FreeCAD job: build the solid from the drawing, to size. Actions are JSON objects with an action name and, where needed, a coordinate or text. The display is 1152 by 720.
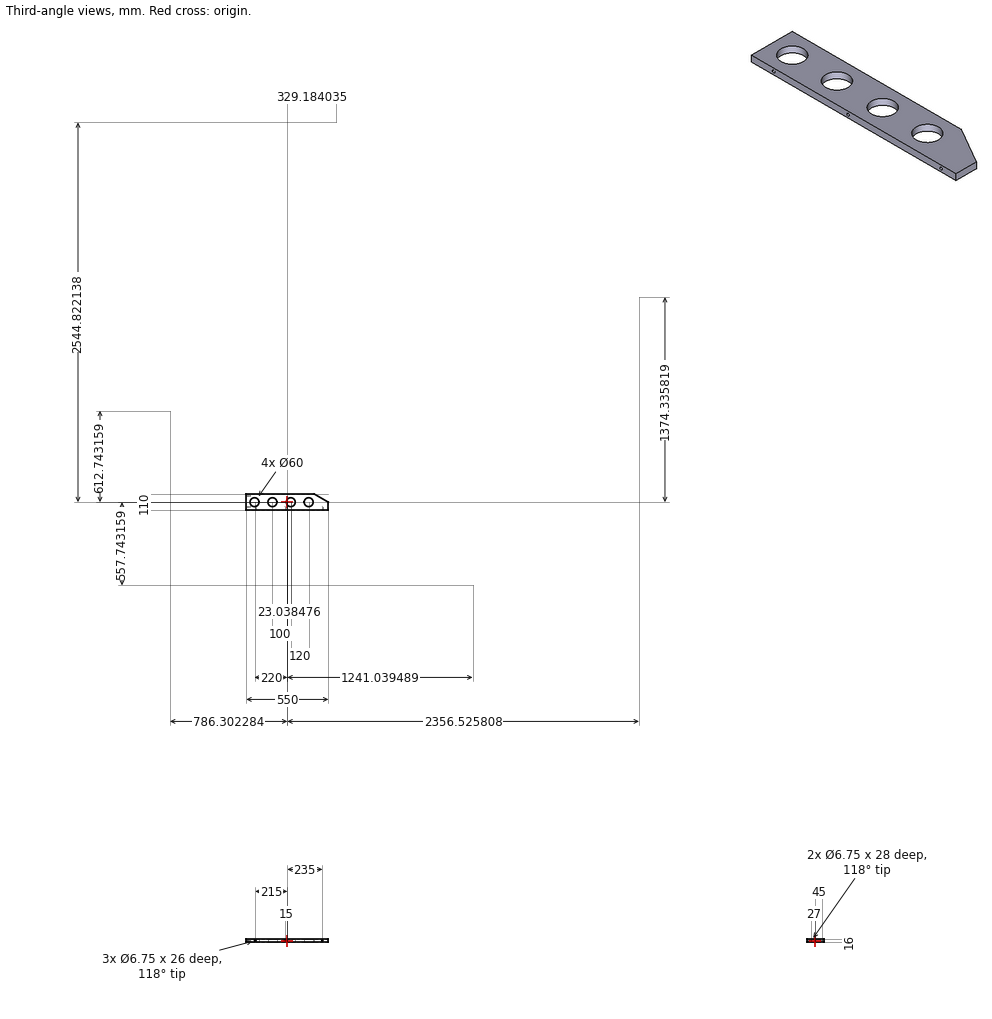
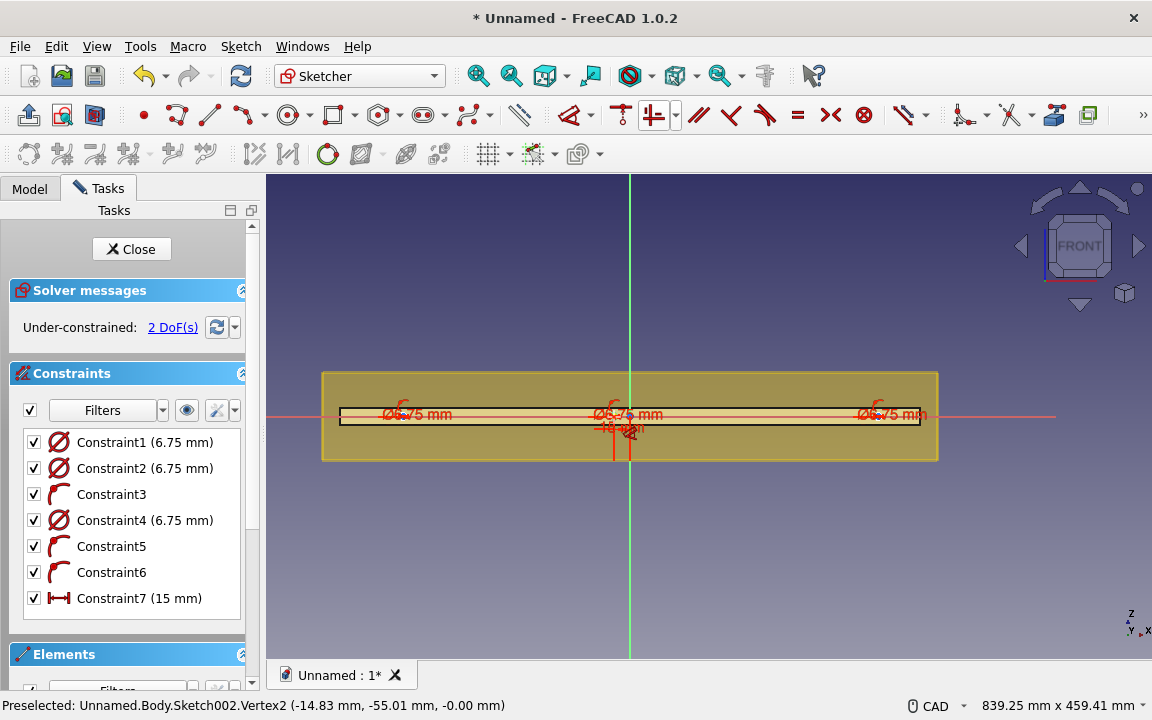
{"action": "left_click", "coordinate": [403, 417]}
{"action": "left_click", "coordinate": [517, 451]}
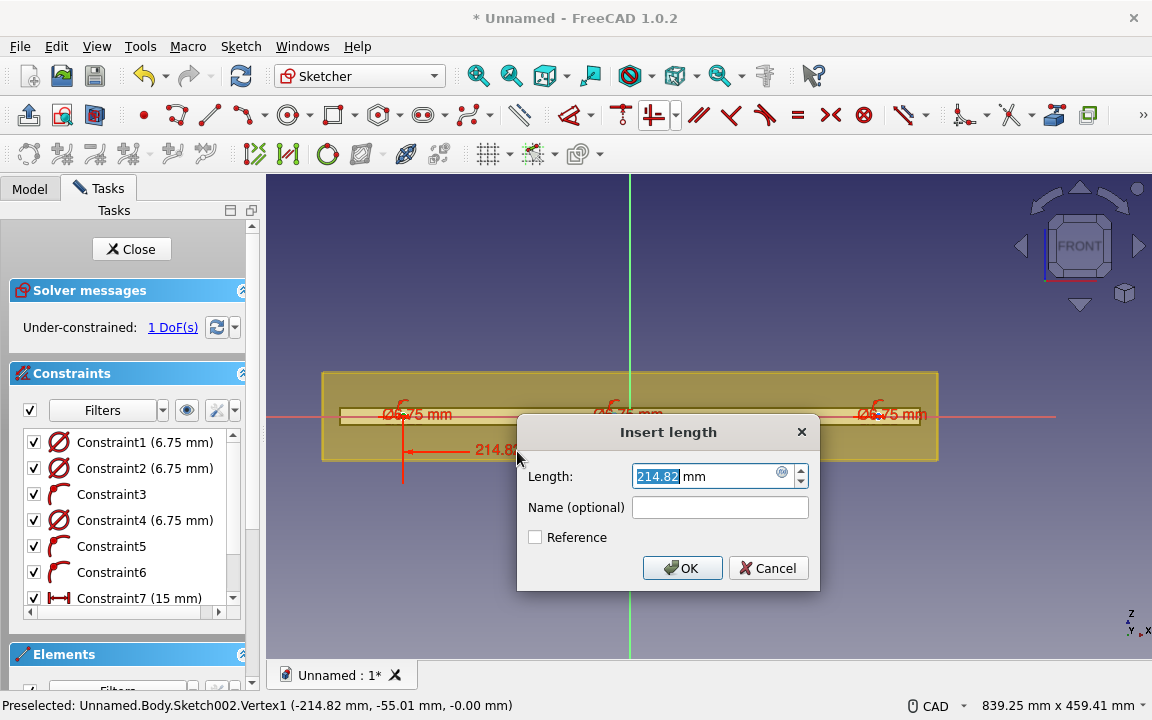
{"action": "type", "text": "215"}
{"action": "key", "text": "Return"}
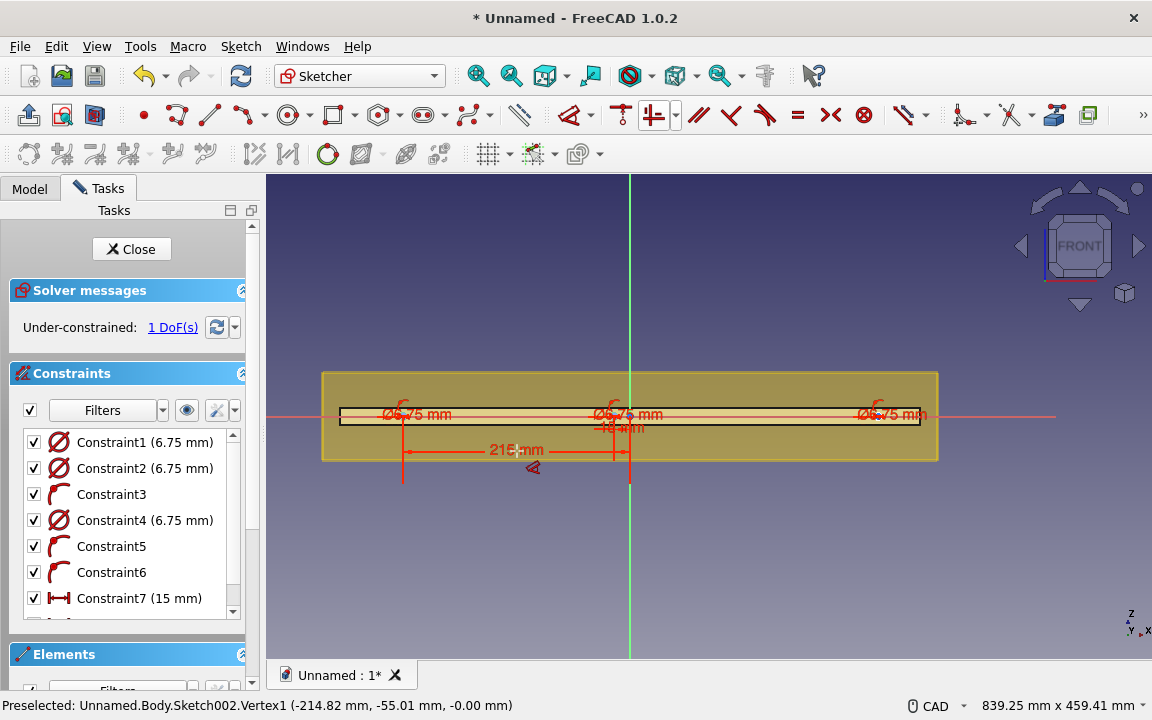
{"action": "left_click", "coordinate": [878, 417]}
{"action": "left_click", "coordinate": [754, 451]}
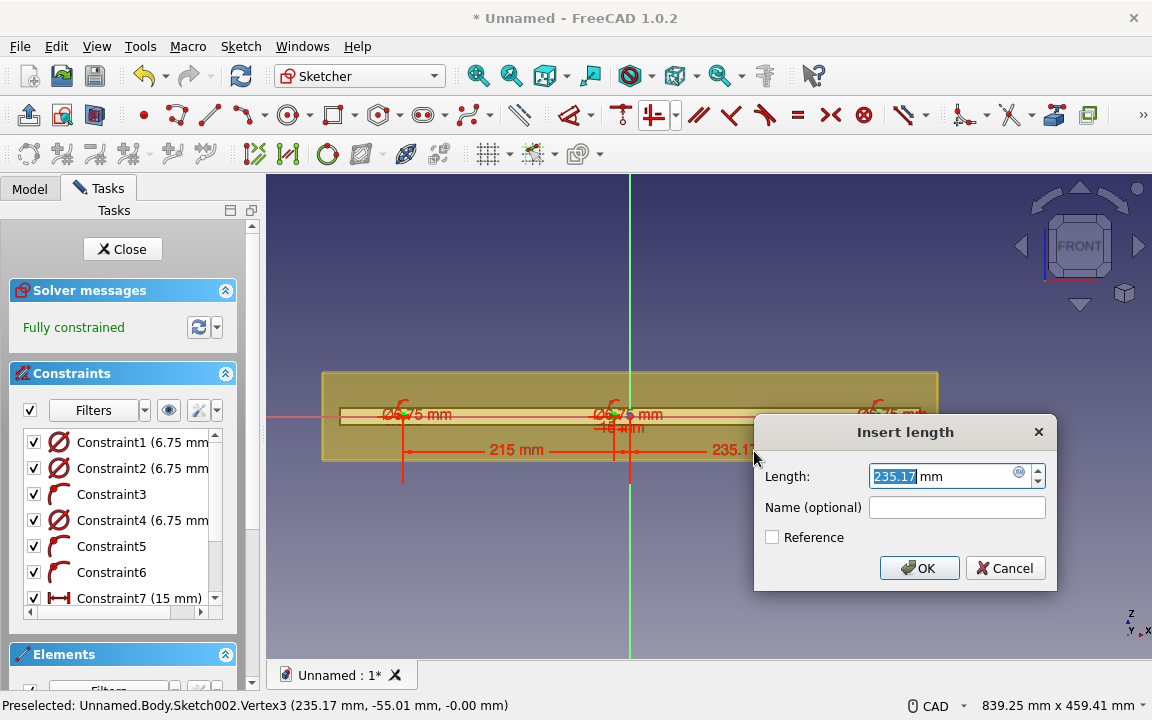
{"action": "type", "text": "235"}
{"action": "key", "text": "Return"}
{"action": "key", "text": "Escape"}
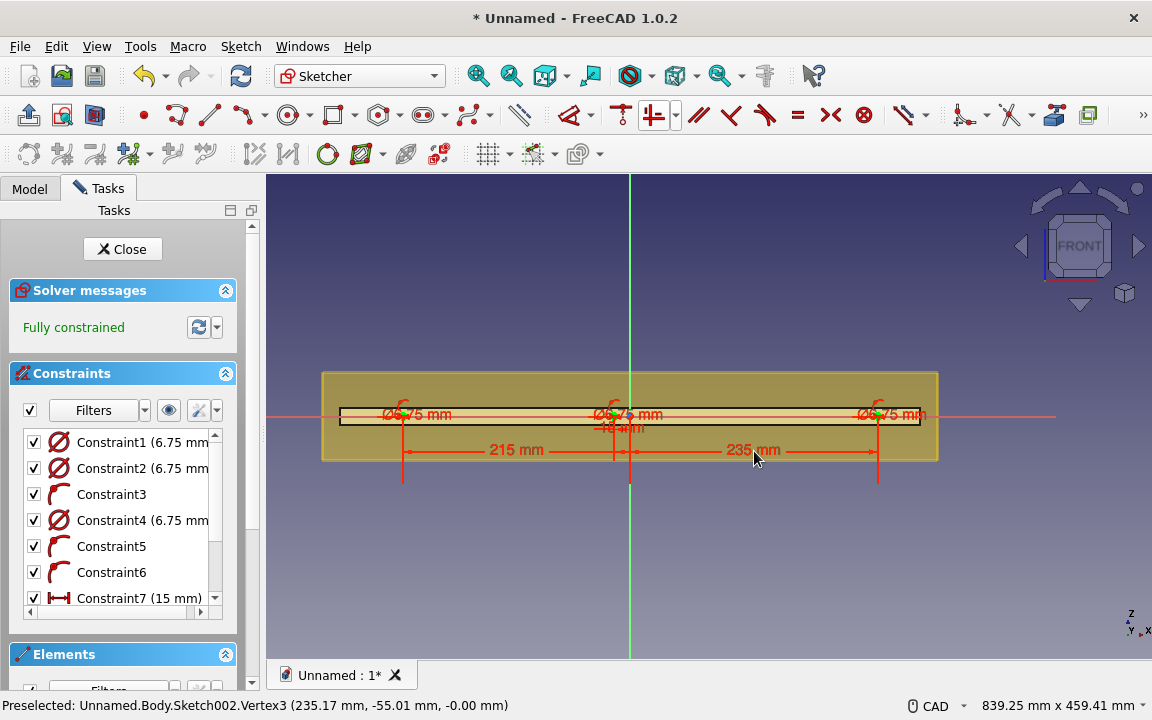
{"action": "left_click", "coordinate": [123, 249]}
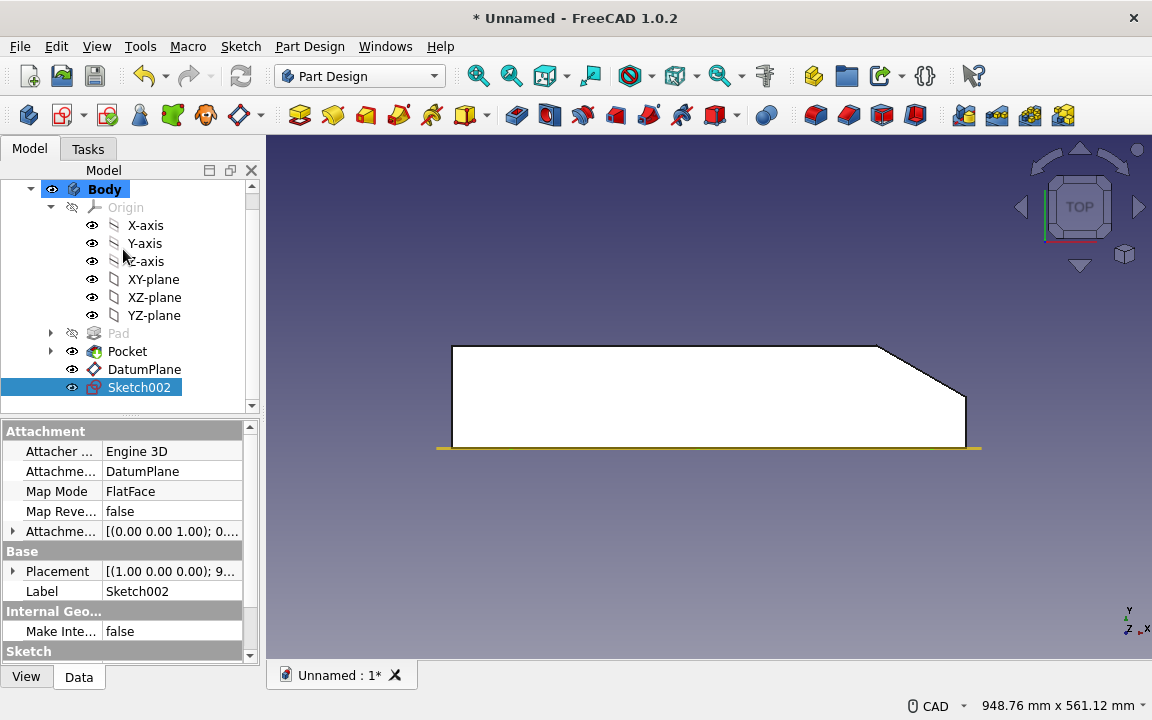
{"action": "left_click", "coordinate": [550, 116]}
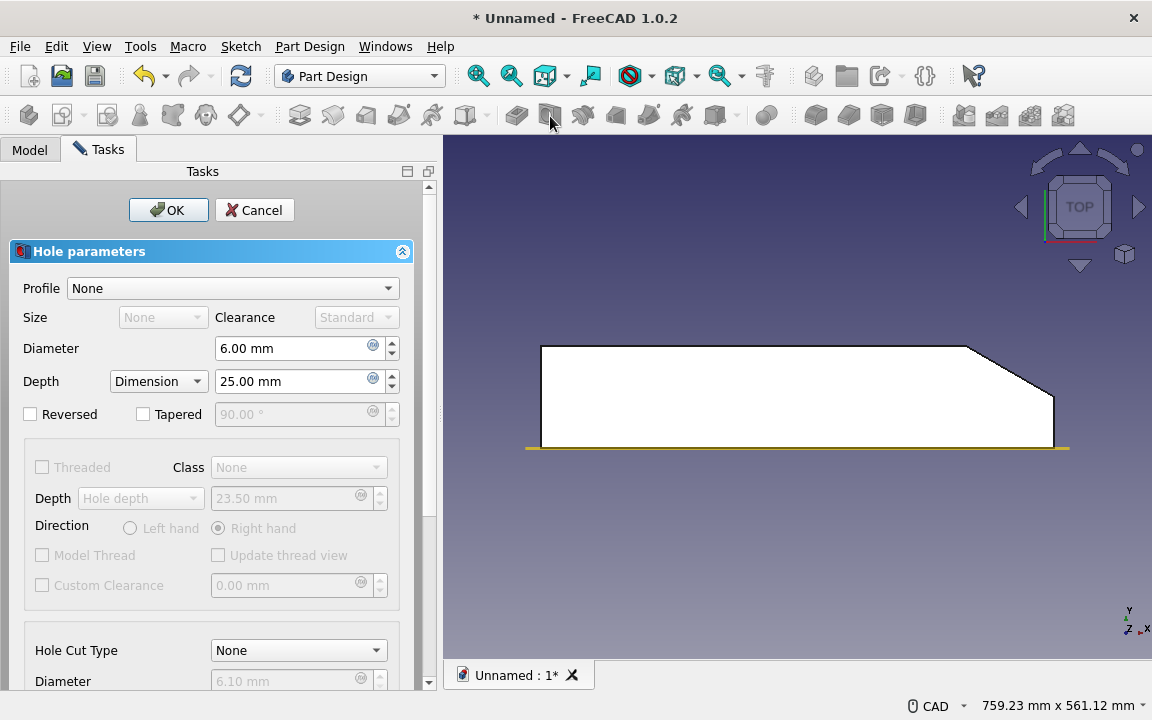
{"action": "triple_click", "coordinate": [300, 348]}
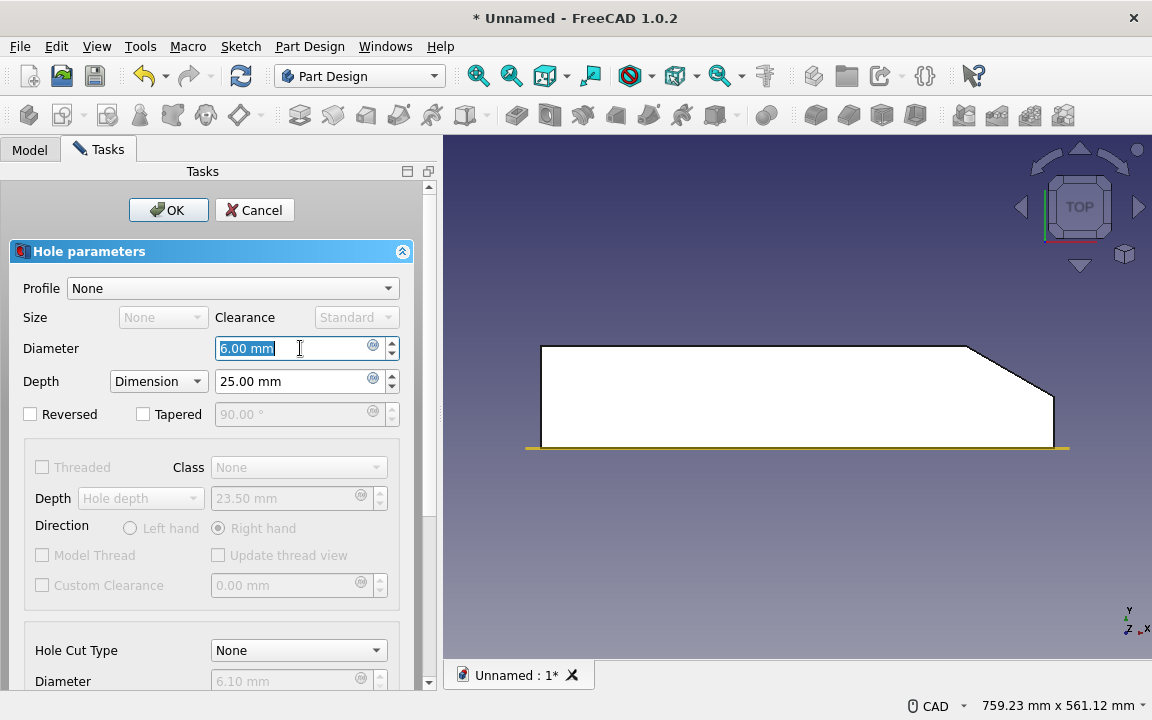
{"action": "type", "text": "6.75"}
{"action": "key", "text": "Tab"}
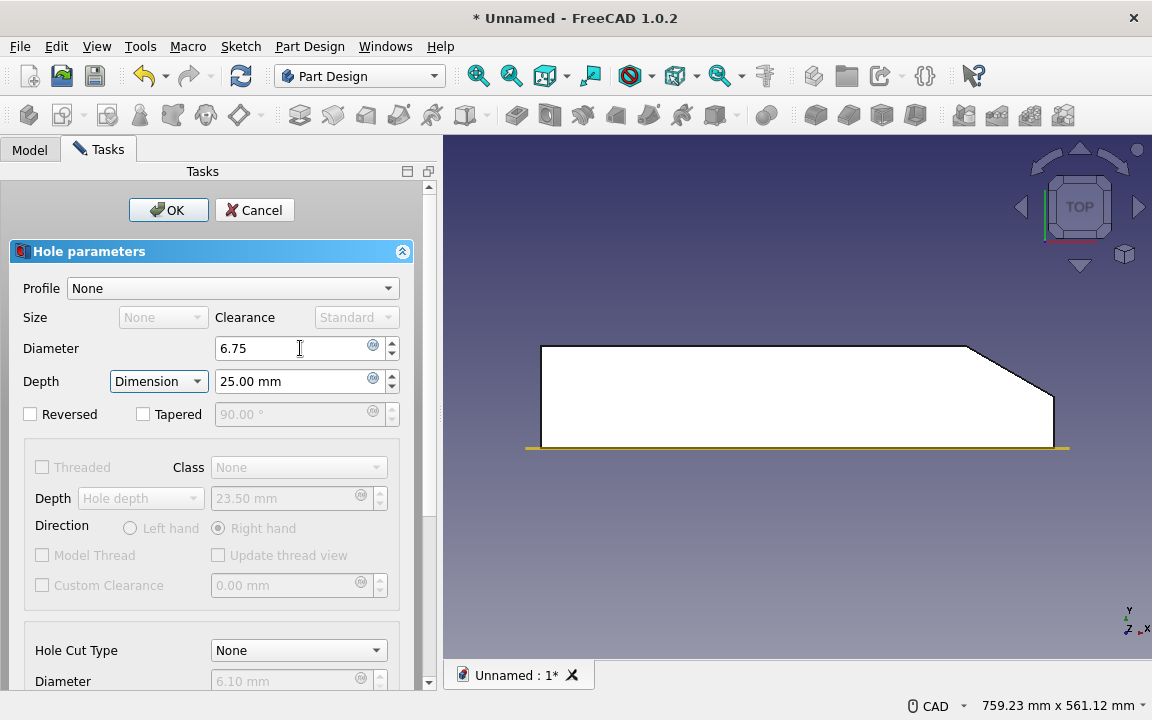
{"action": "triple_click", "coordinate": [300, 382]}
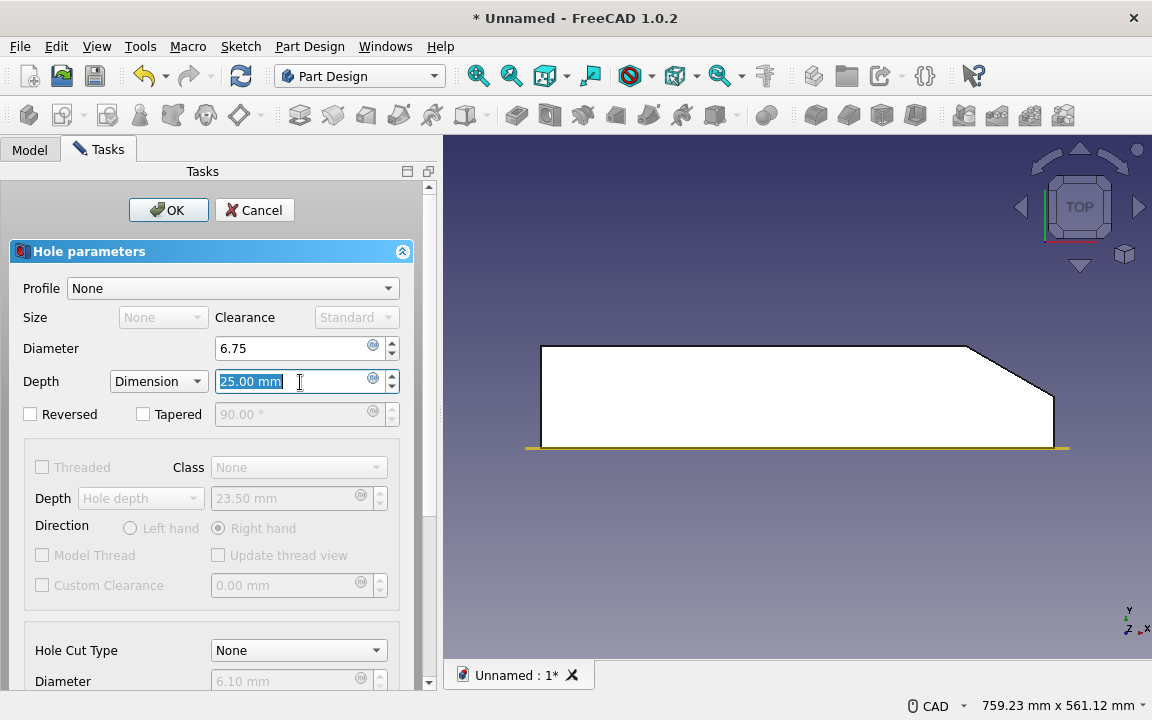
{"action": "type", "text": "26"}
{"action": "key", "text": "Tab"}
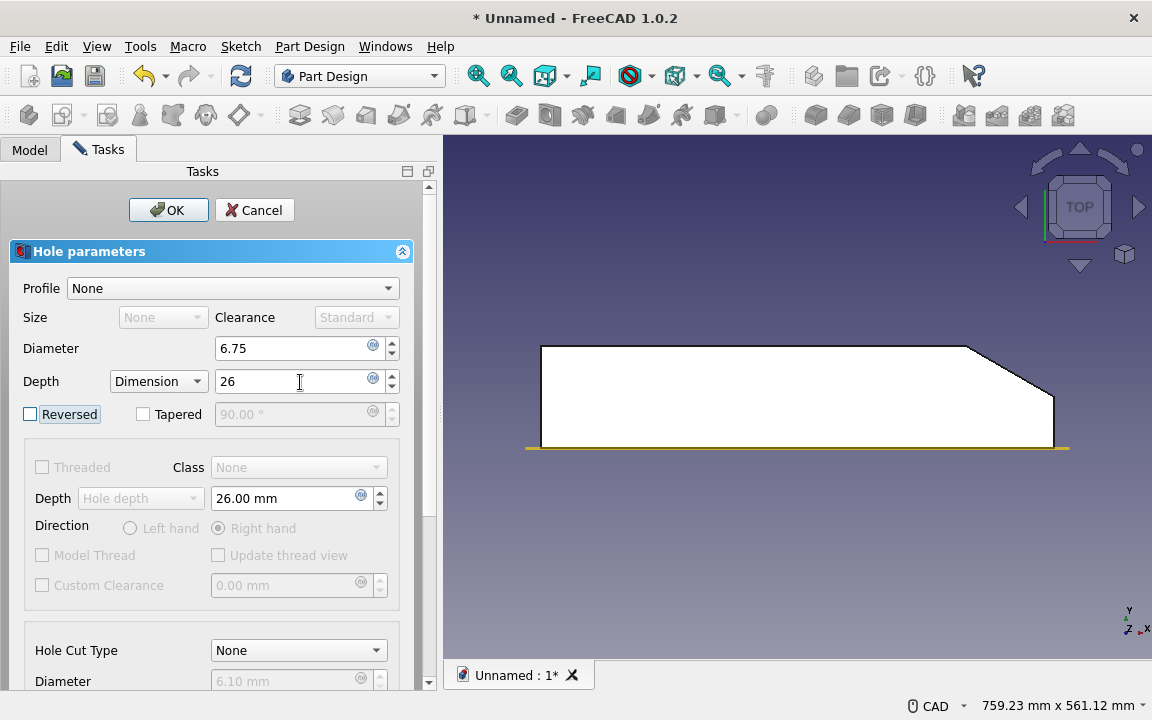
{"action": "left_click", "coordinate": [169, 210]}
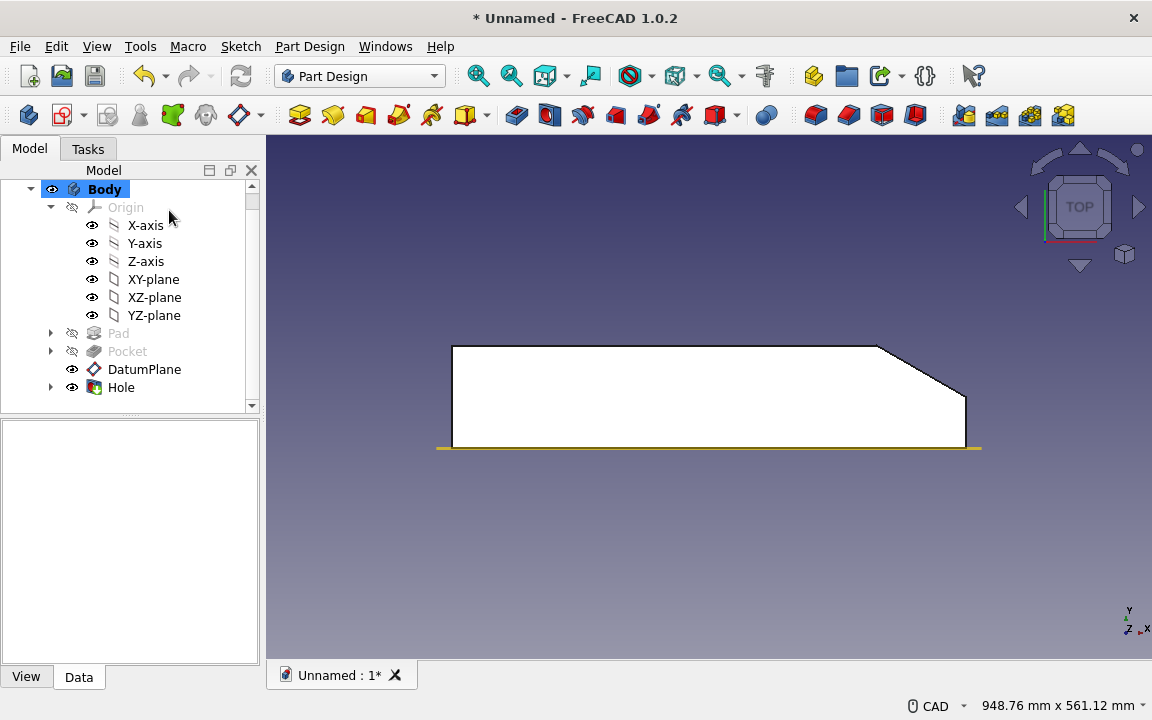
{"action": "left_click", "coordinate": [117, 369]}
{"action": "key", "text": "space"}